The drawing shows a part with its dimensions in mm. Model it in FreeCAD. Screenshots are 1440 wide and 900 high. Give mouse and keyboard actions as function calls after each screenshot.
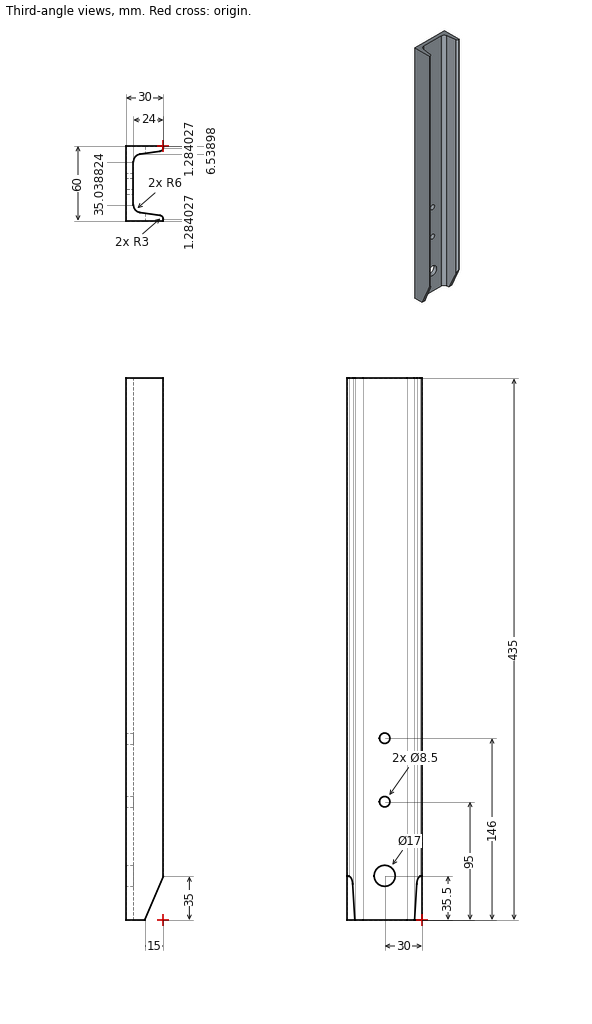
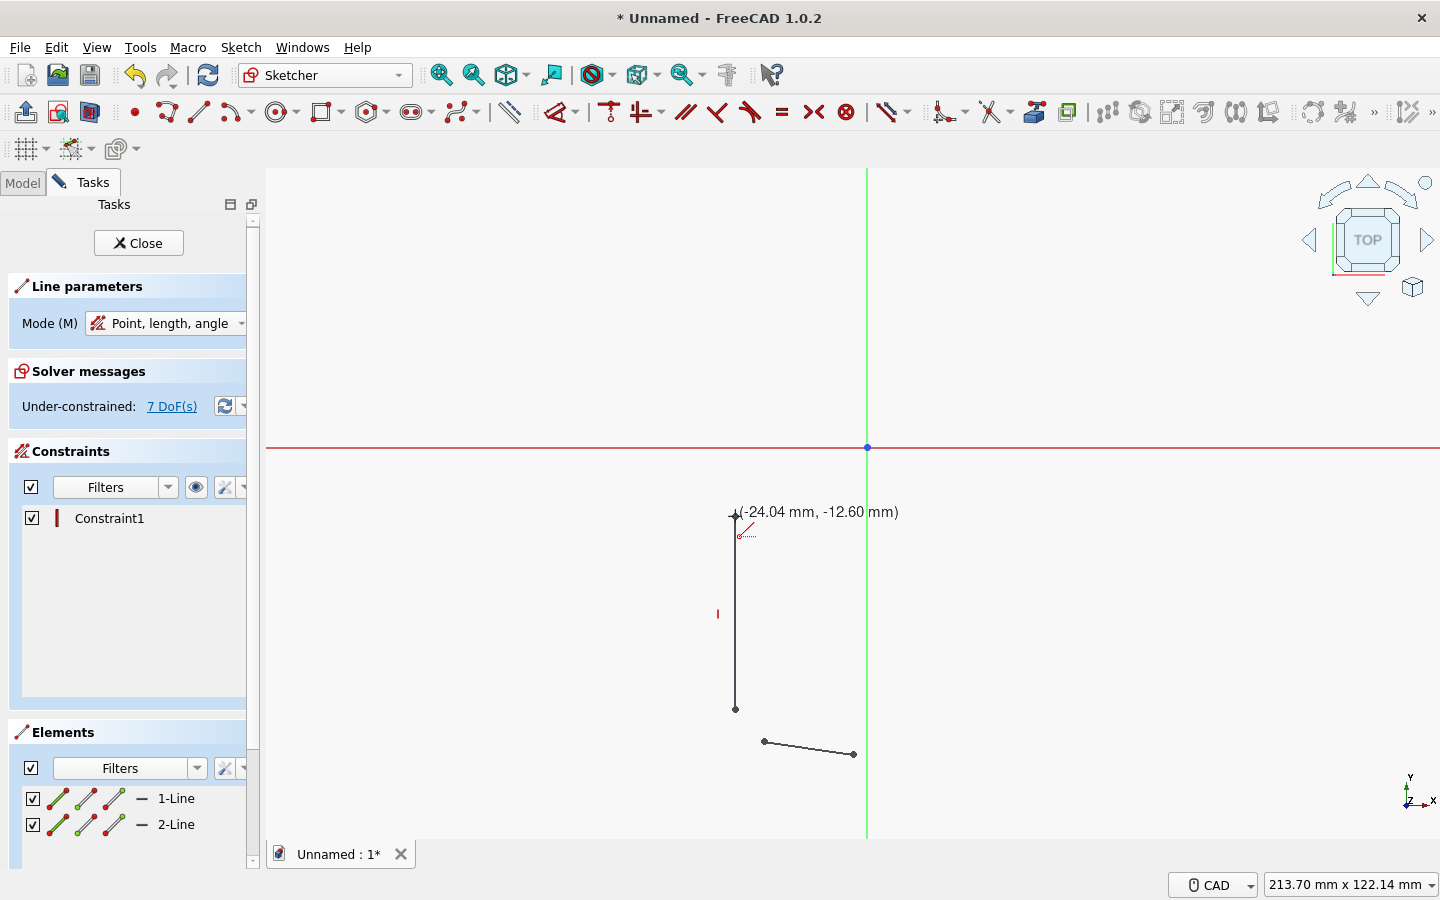
click(764, 484)
click(853, 471)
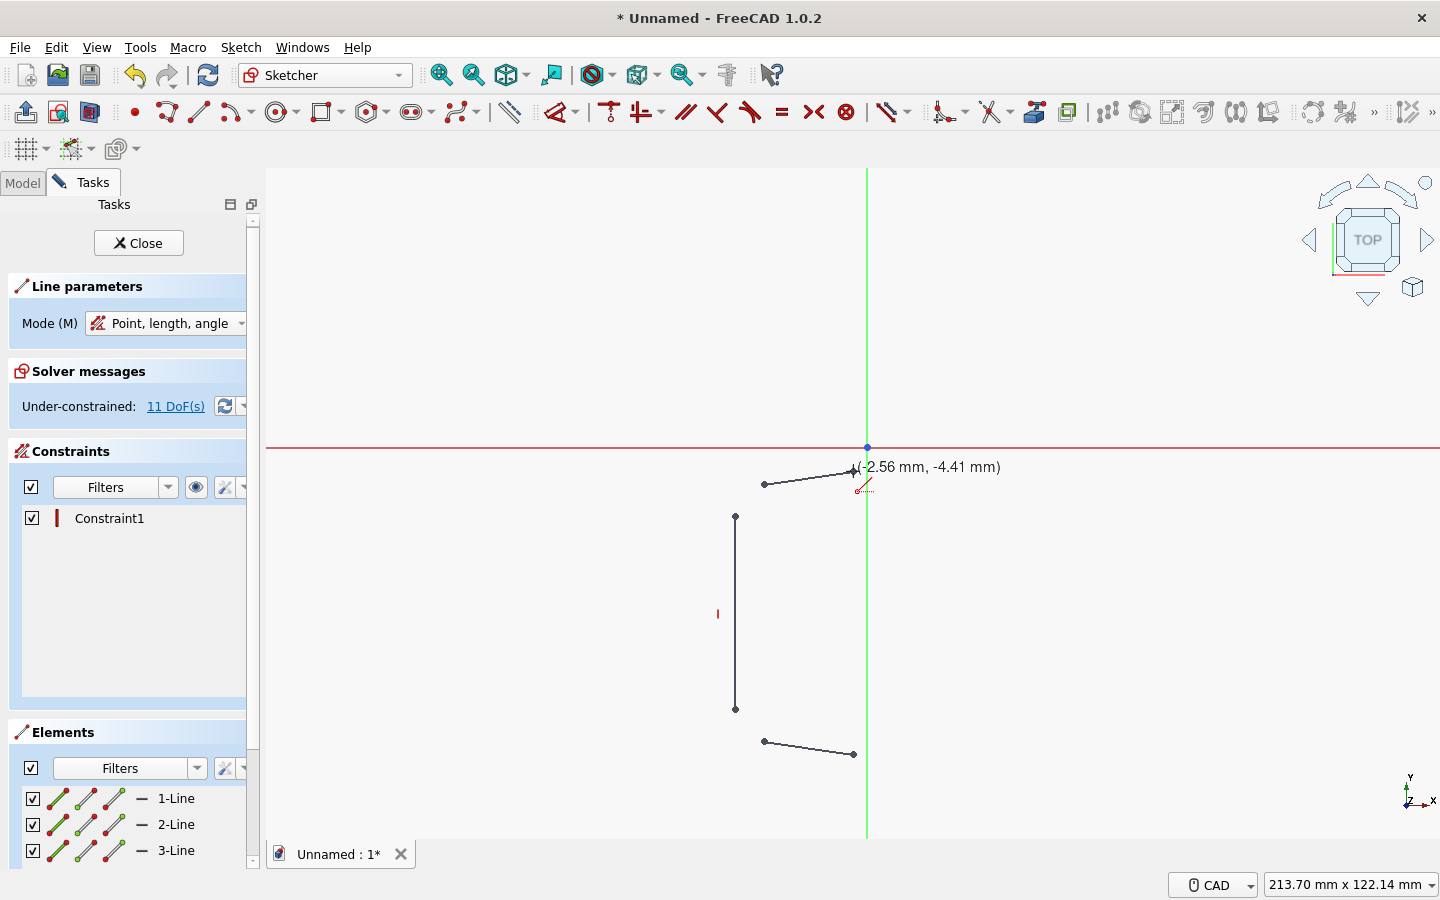
click(168, 112)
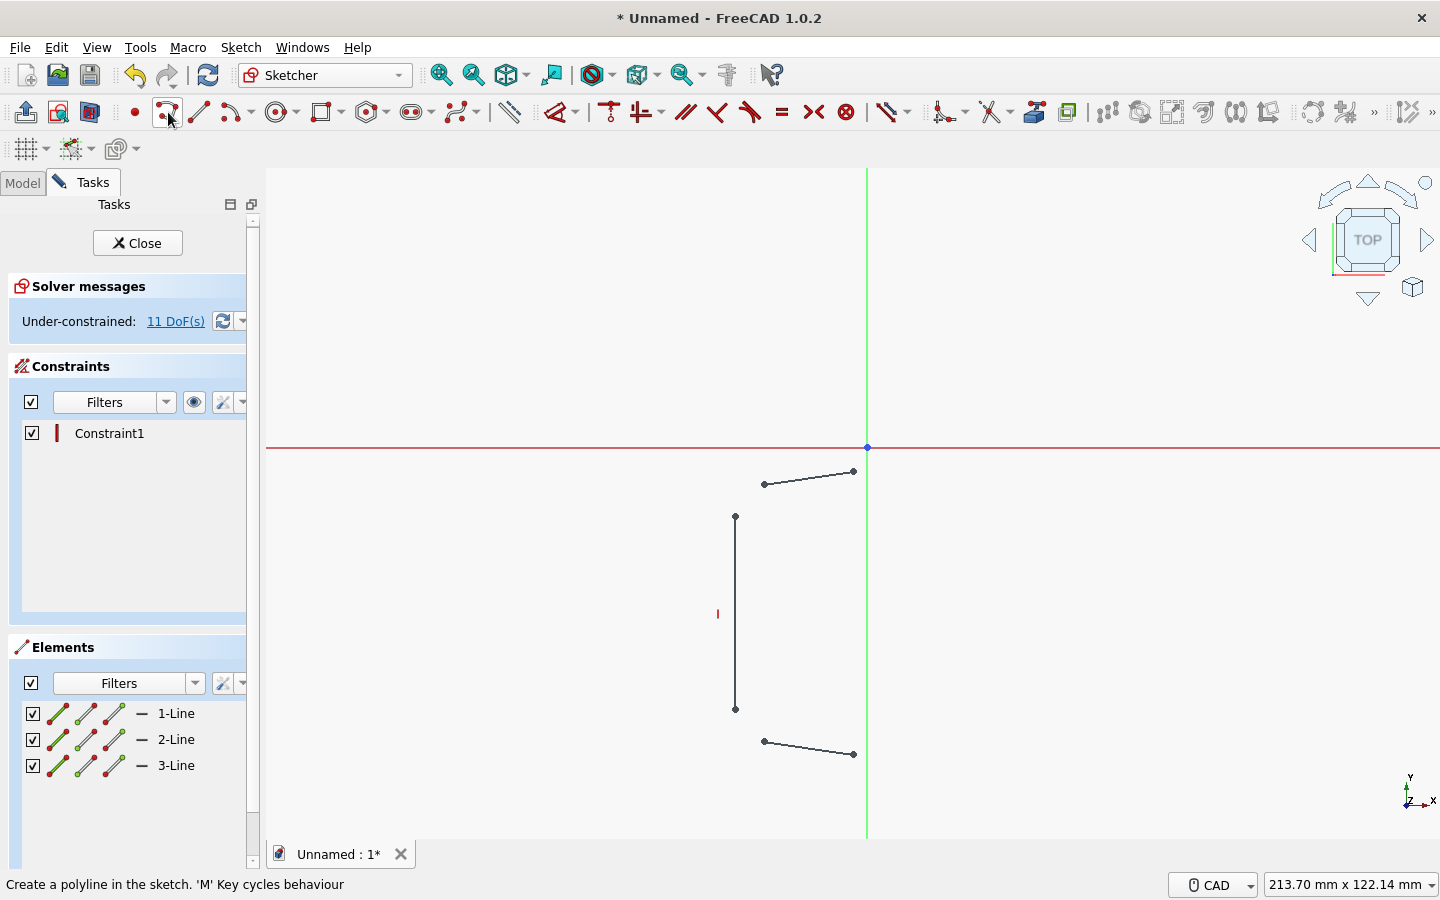
scroll(867, 455, up, 5)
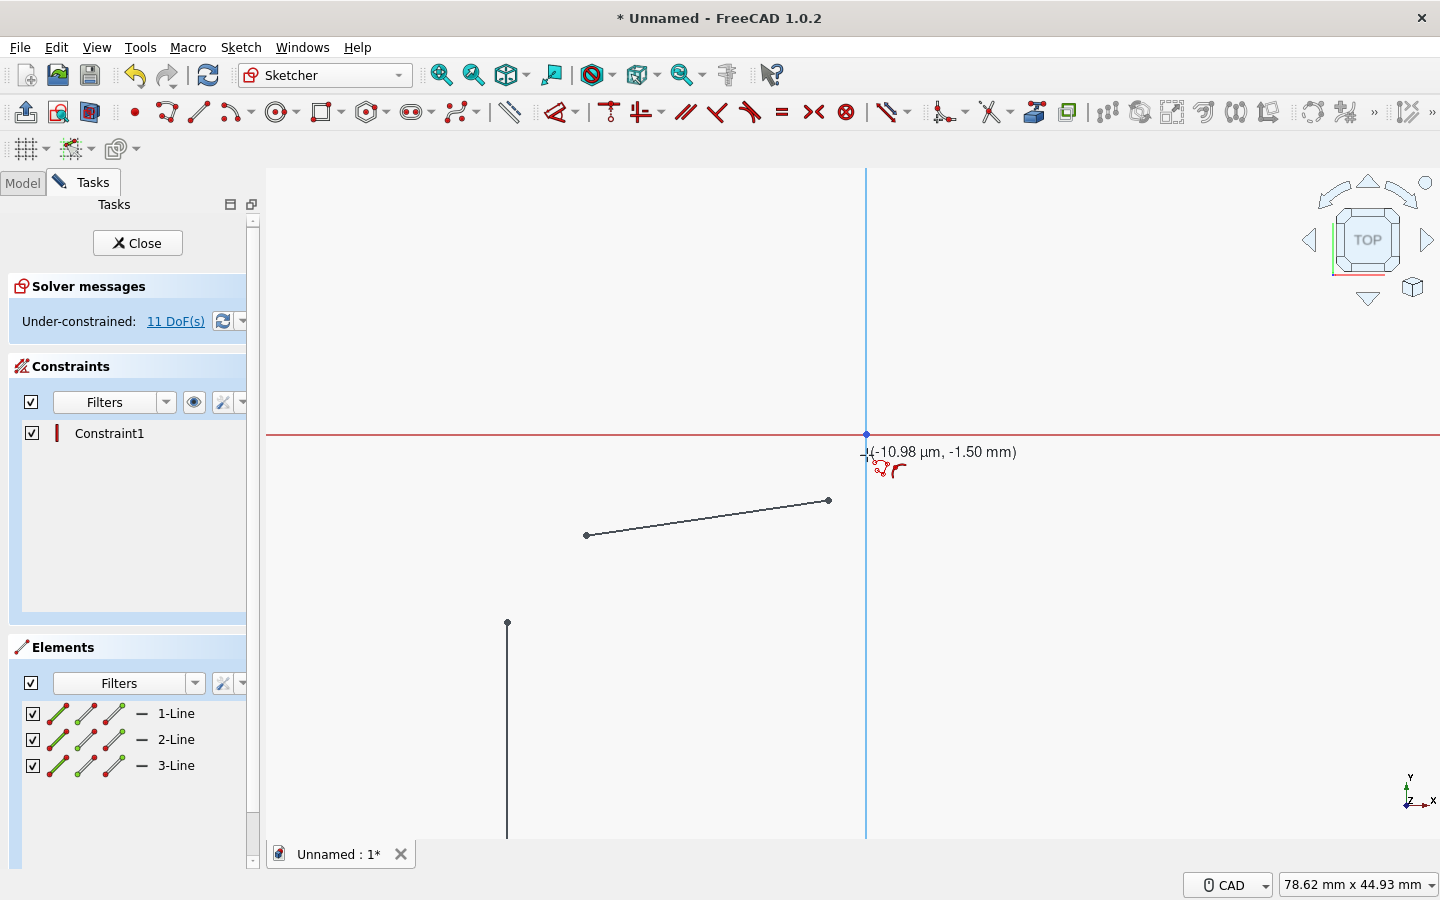
click(866, 454)
click(866, 435)
click(418, 444)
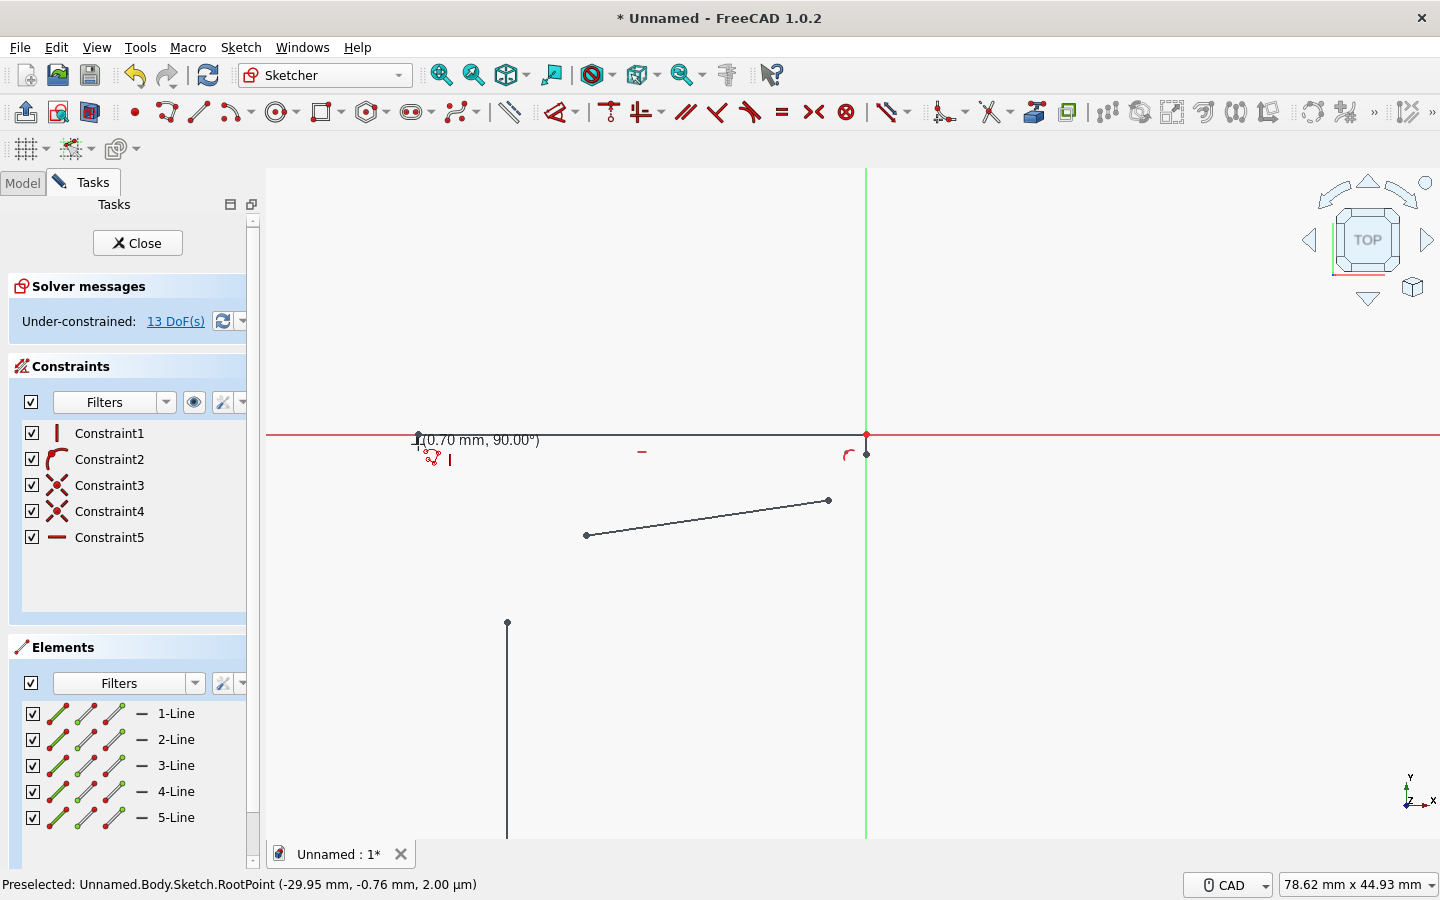
scroll(901, 196, down, 4)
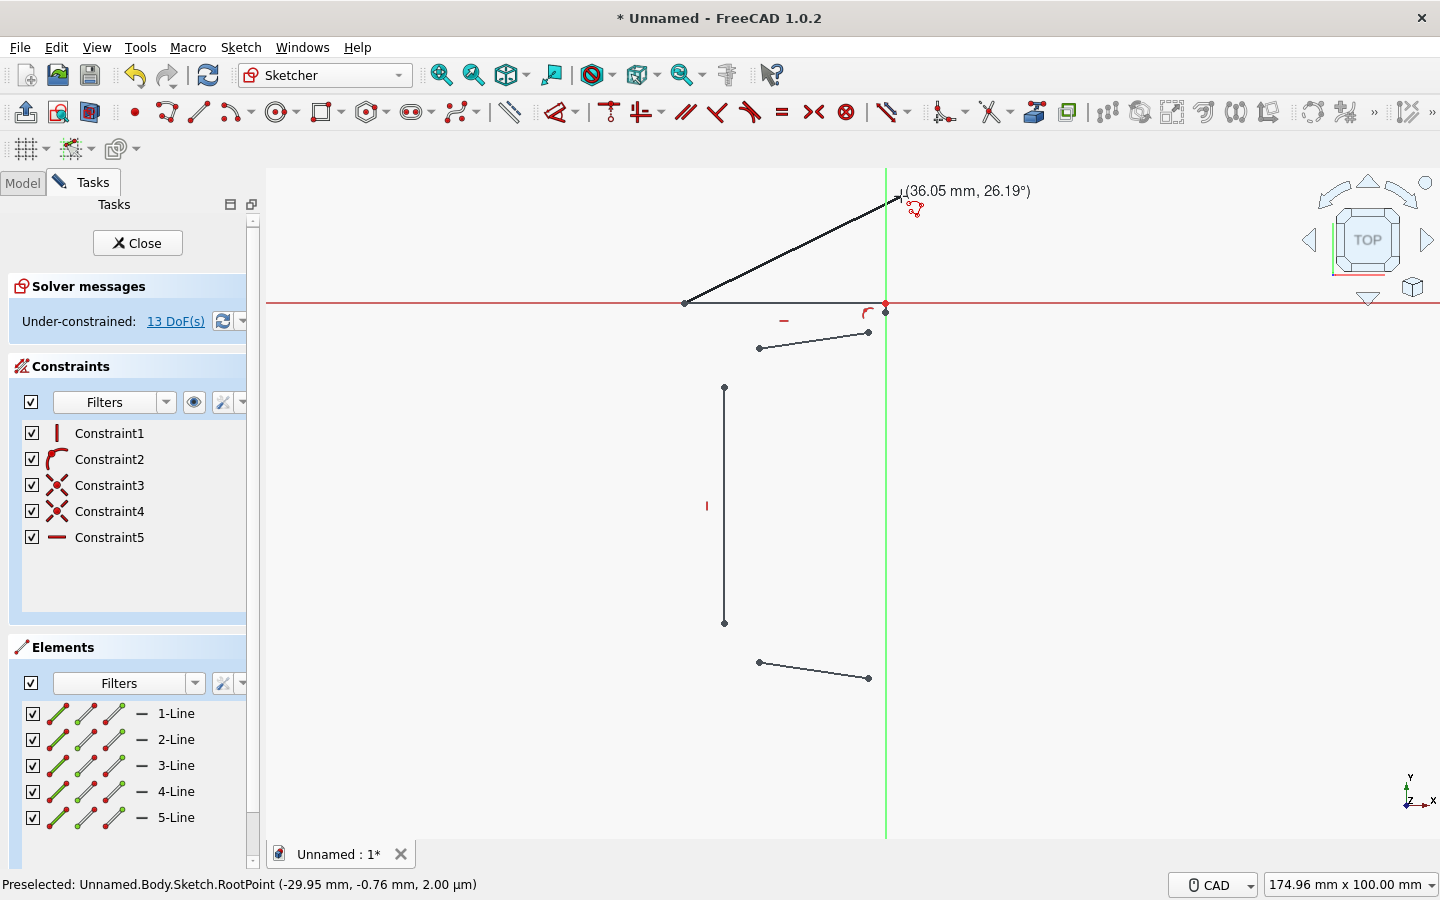
click(684, 706)
click(886, 706)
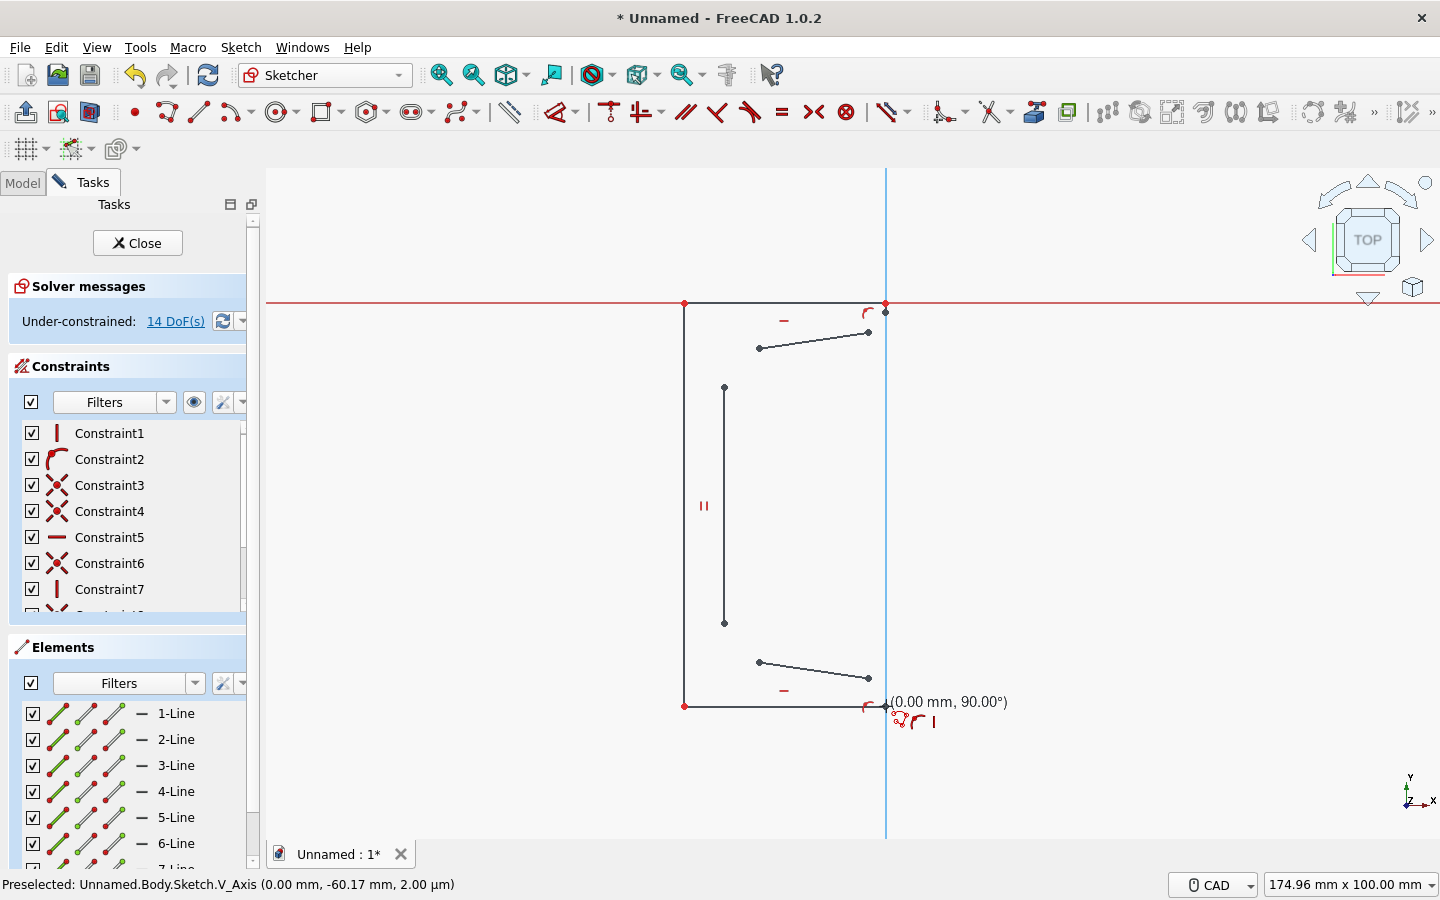
scroll(886, 697, up, 4)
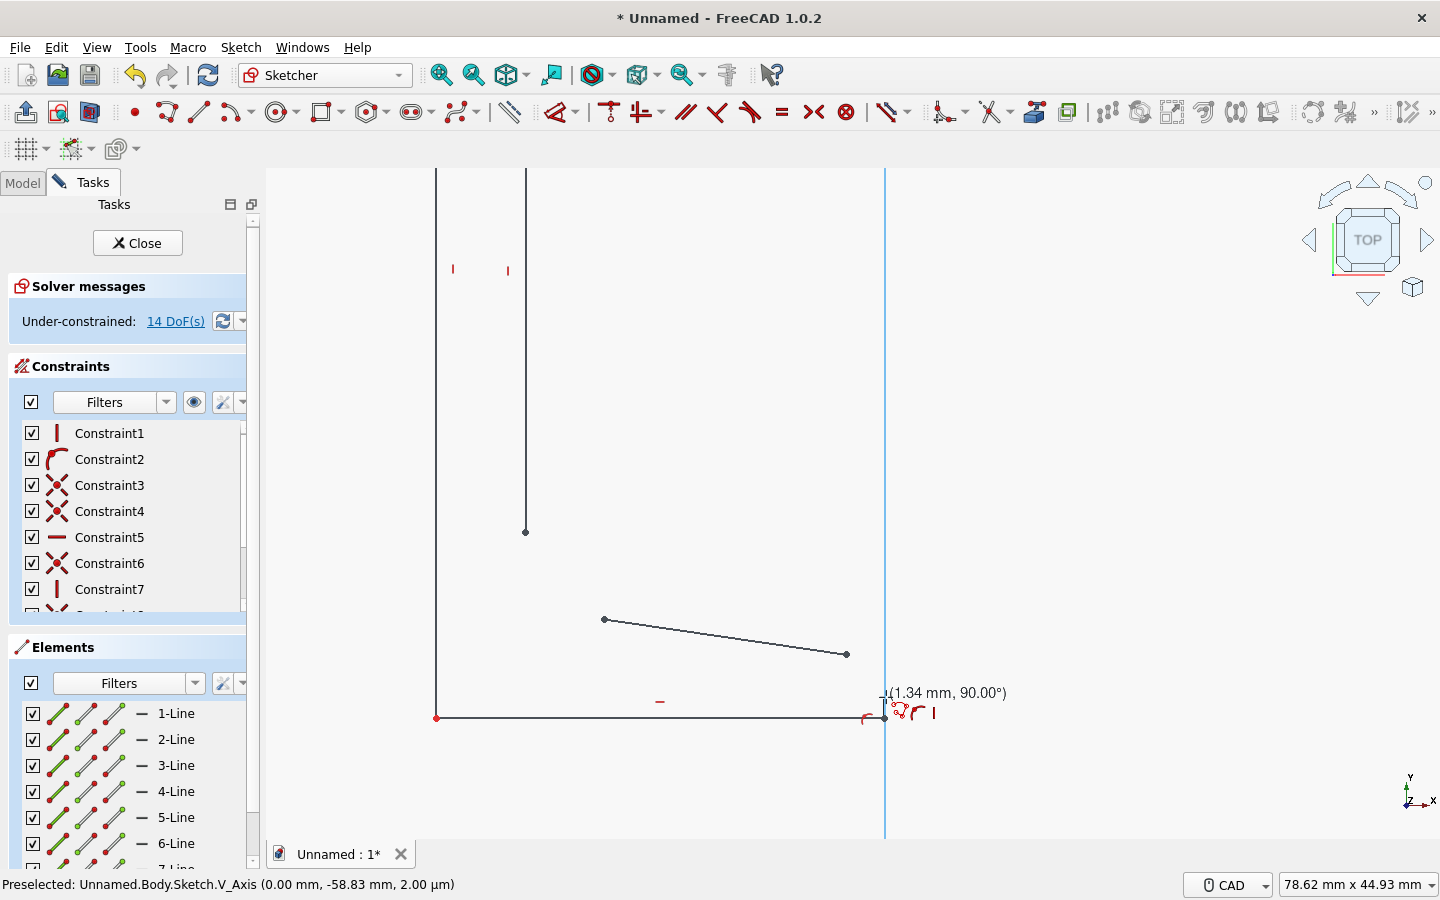
click(876, 697)
right_click(876, 697)